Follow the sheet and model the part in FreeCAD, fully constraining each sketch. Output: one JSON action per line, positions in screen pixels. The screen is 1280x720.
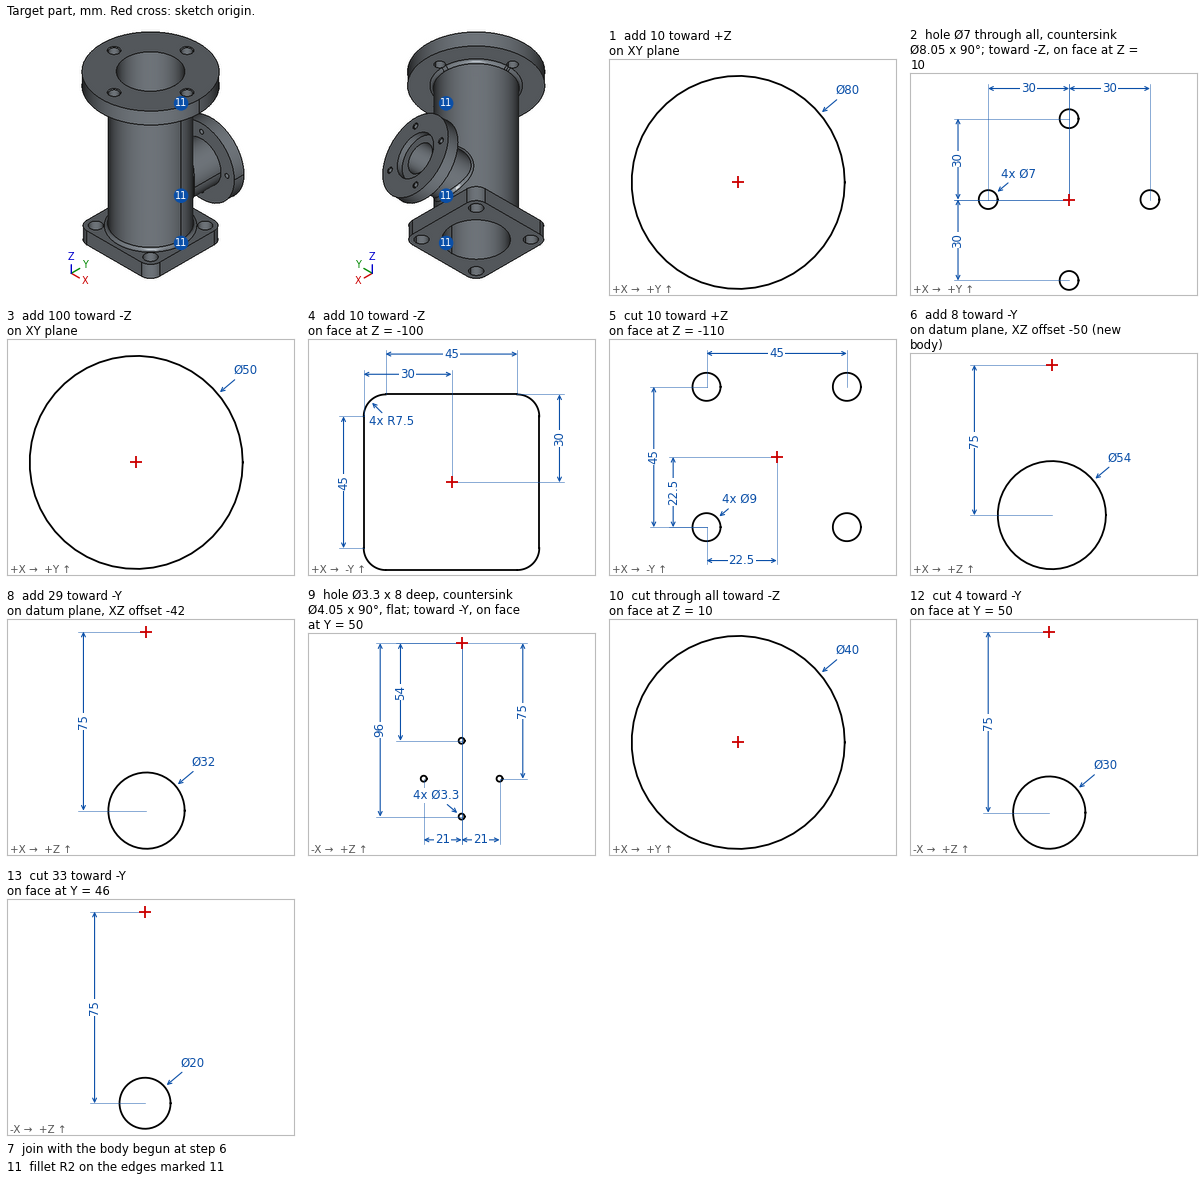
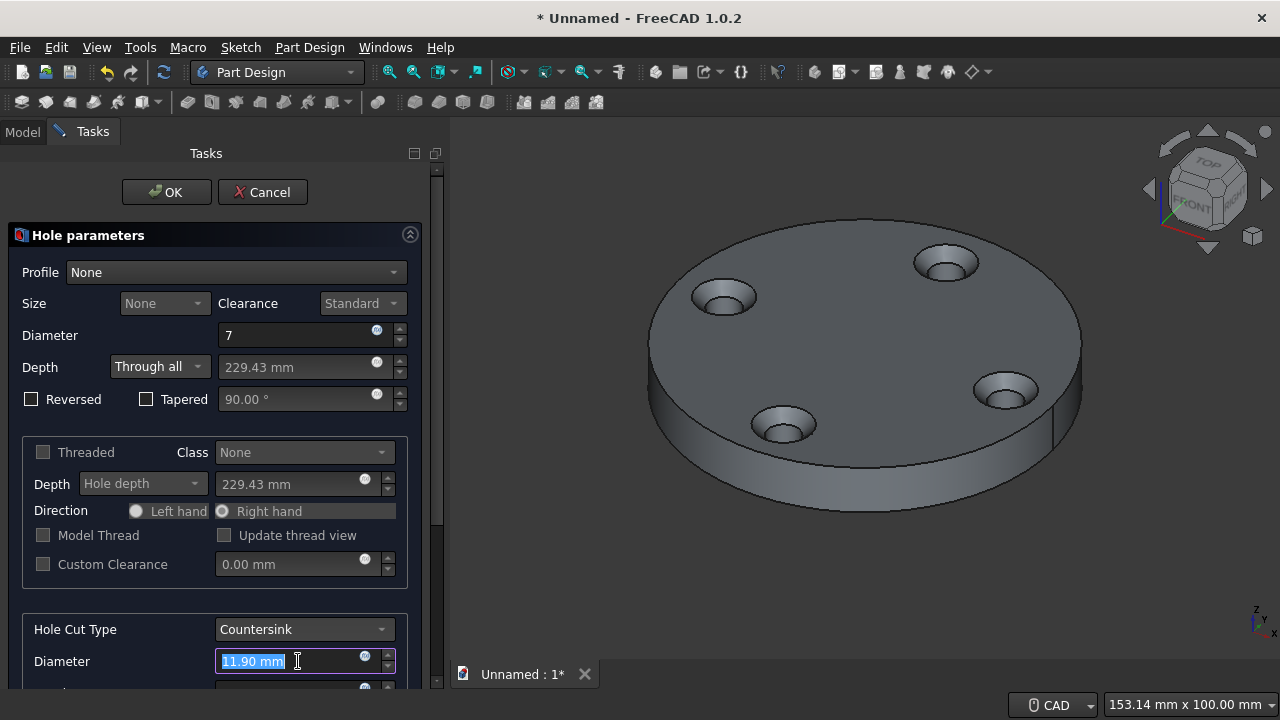
{"action": "type", "text": "8.05"}
{"action": "key", "text": "Tab"}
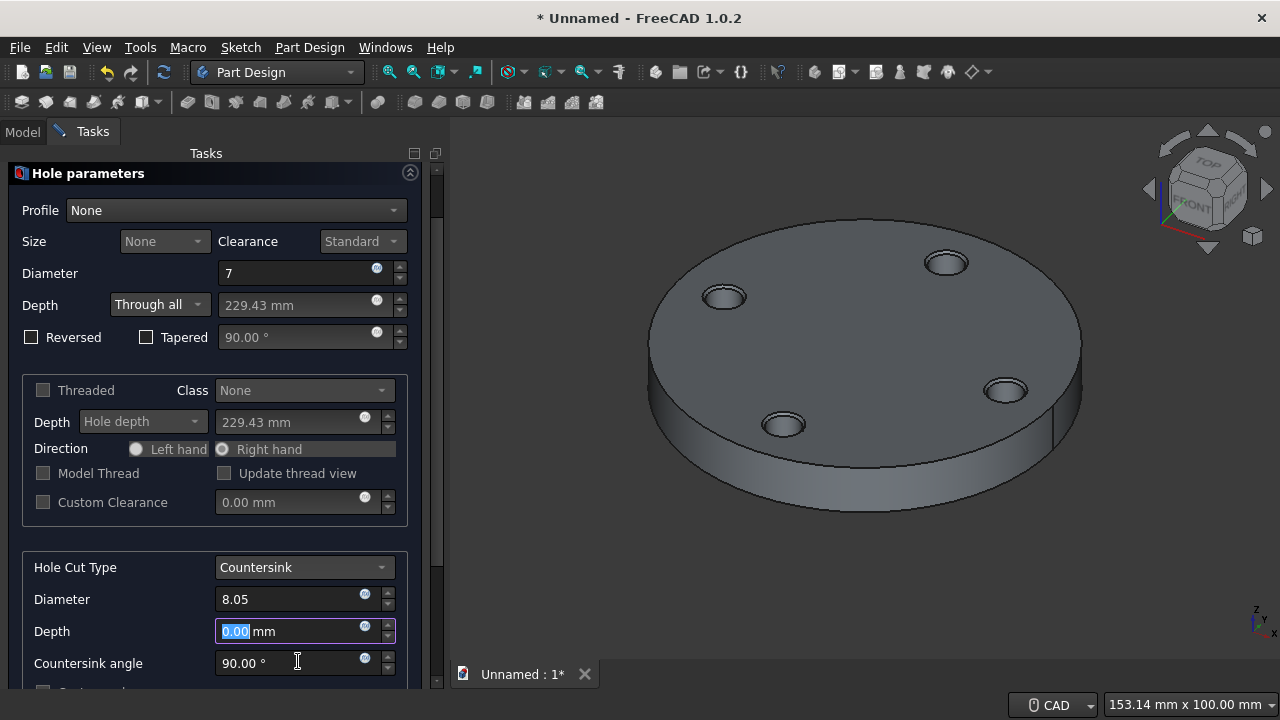
{"action": "scroll", "coordinate": [437, 426], "scroll_direction": "up", "scroll_amount": 2}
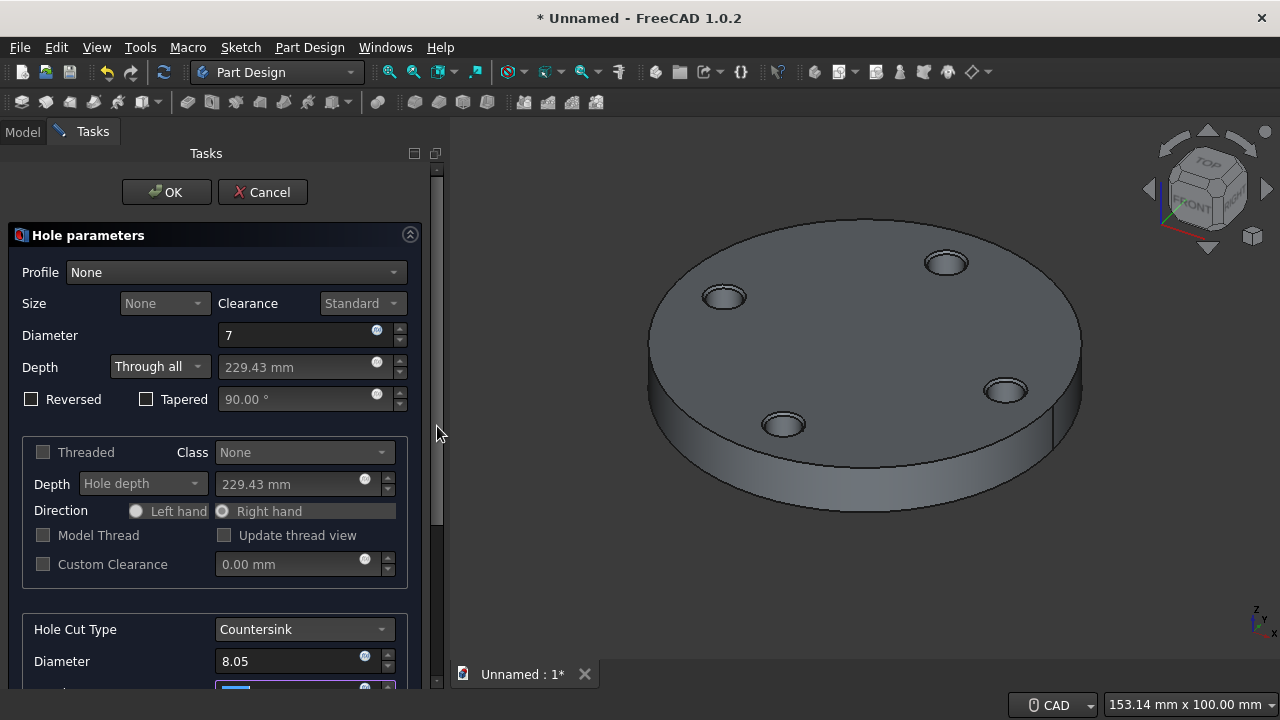
{"action": "left_click", "coordinate": [167, 192]}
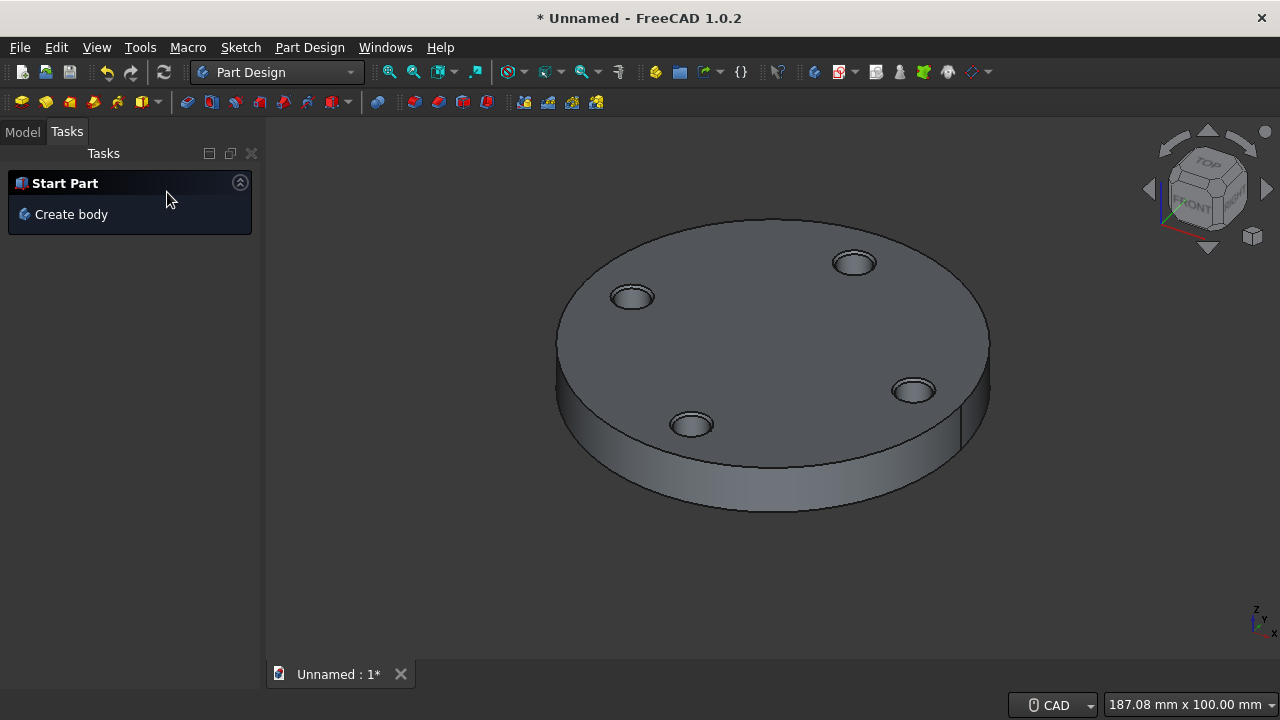
{"action": "left_click", "coordinate": [840, 72]}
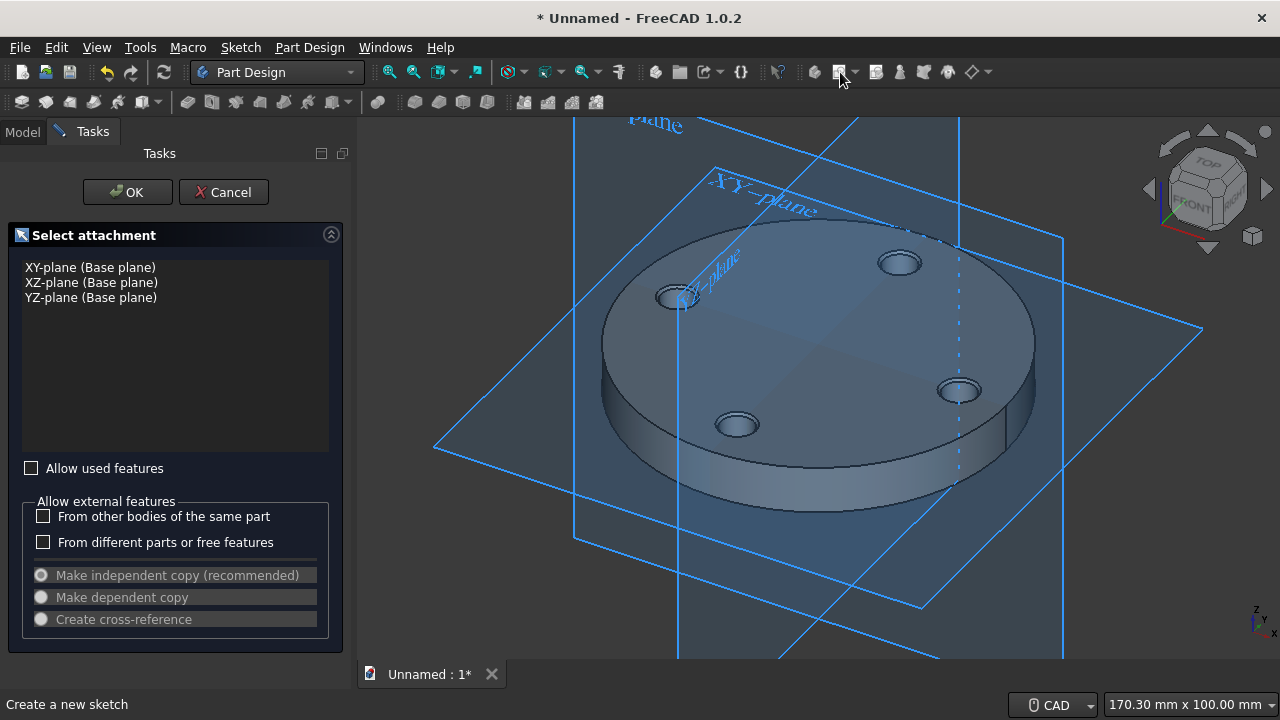
{"action": "left_click", "coordinate": [82, 268]}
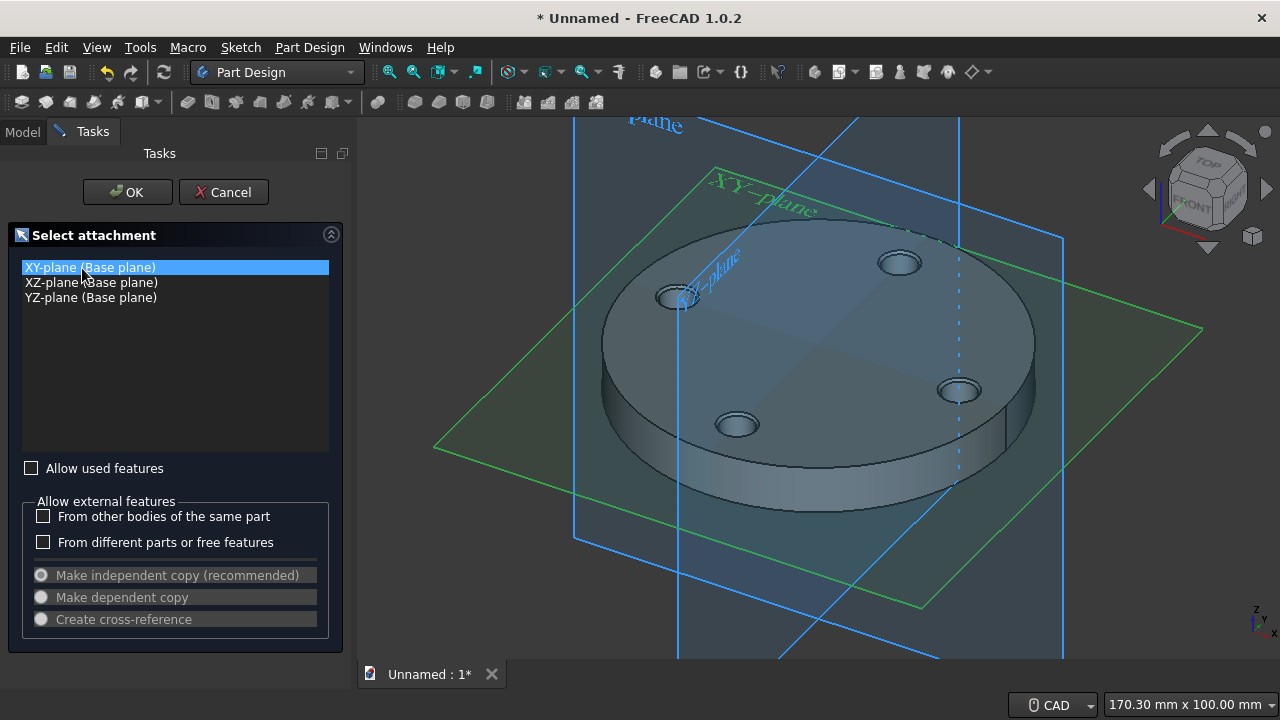
{"action": "left_click", "coordinate": [128, 192]}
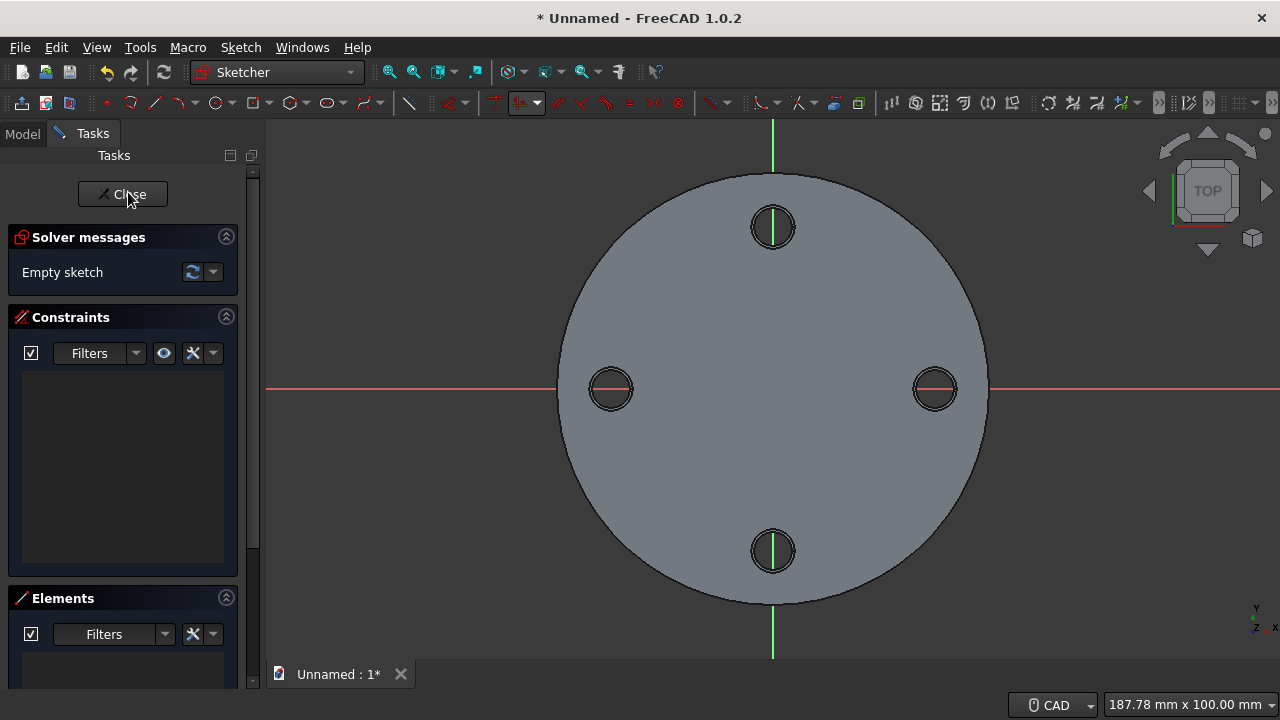
{"action": "left_click", "coordinate": [70, 104]}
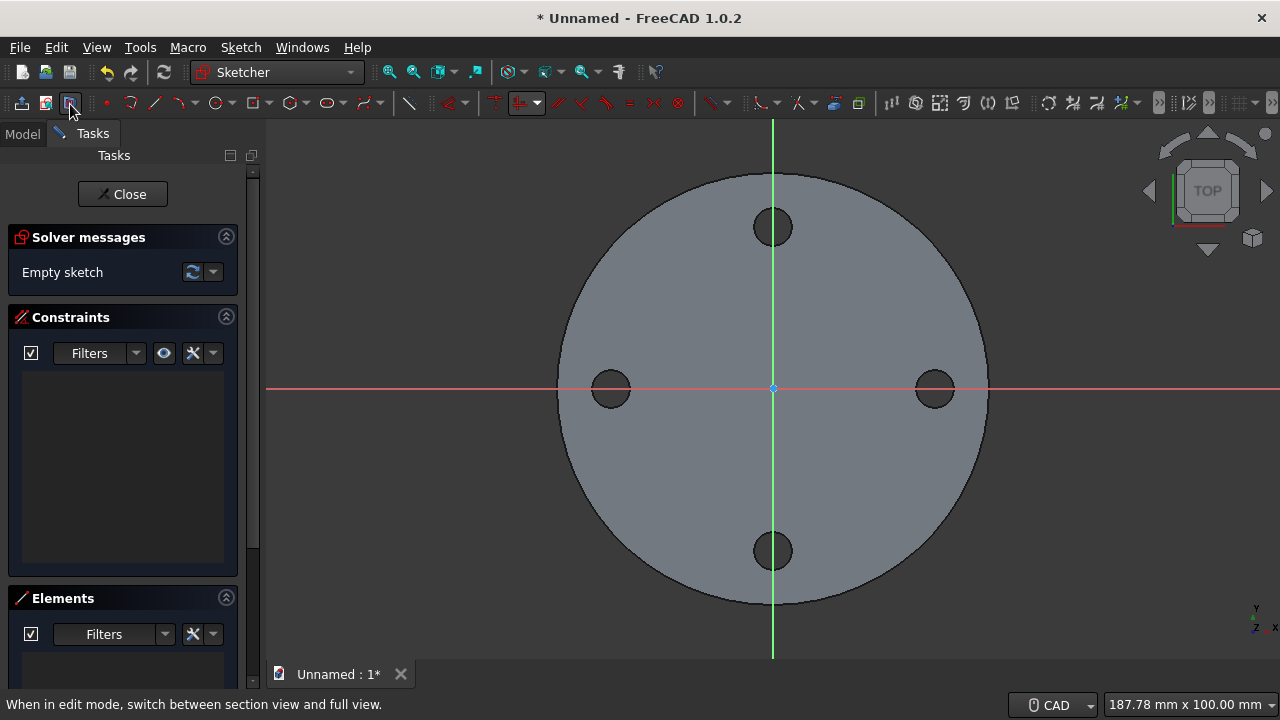
{"action": "left_click", "coordinate": [216, 104]}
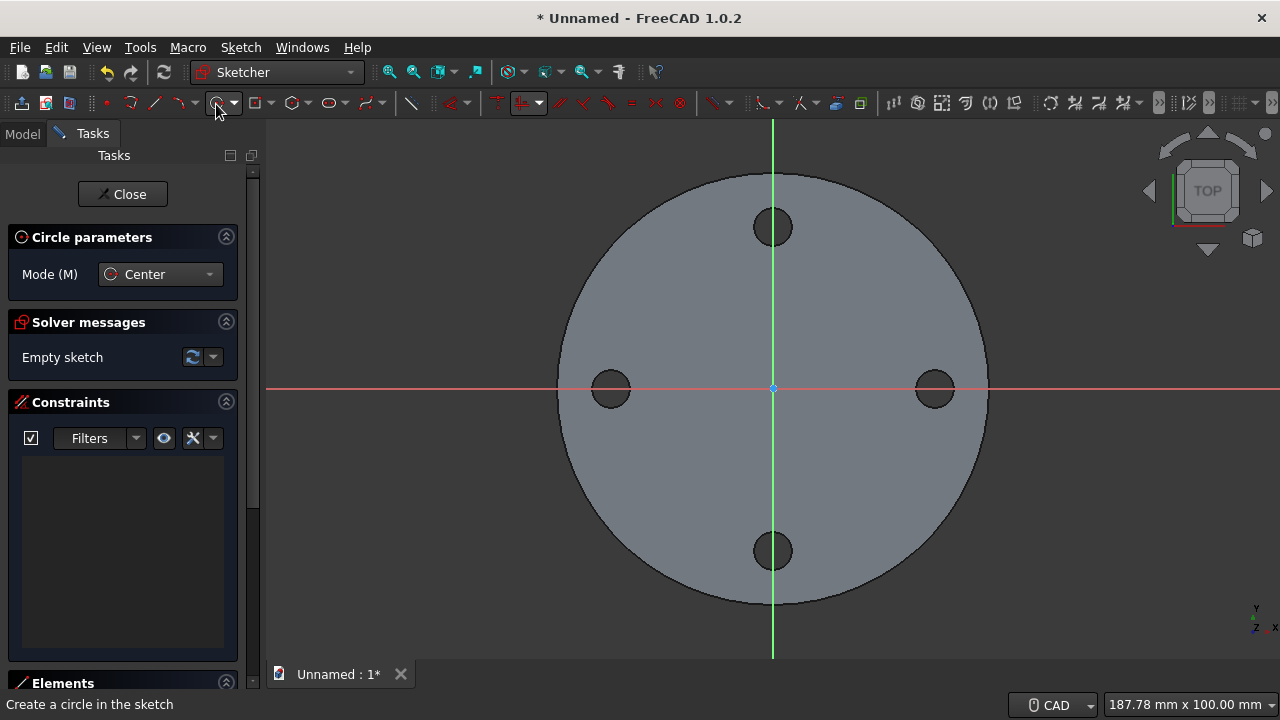
{"action": "left_click", "coordinate": [773, 389]}
{"action": "mouse_move", "coordinate": [868, 294]}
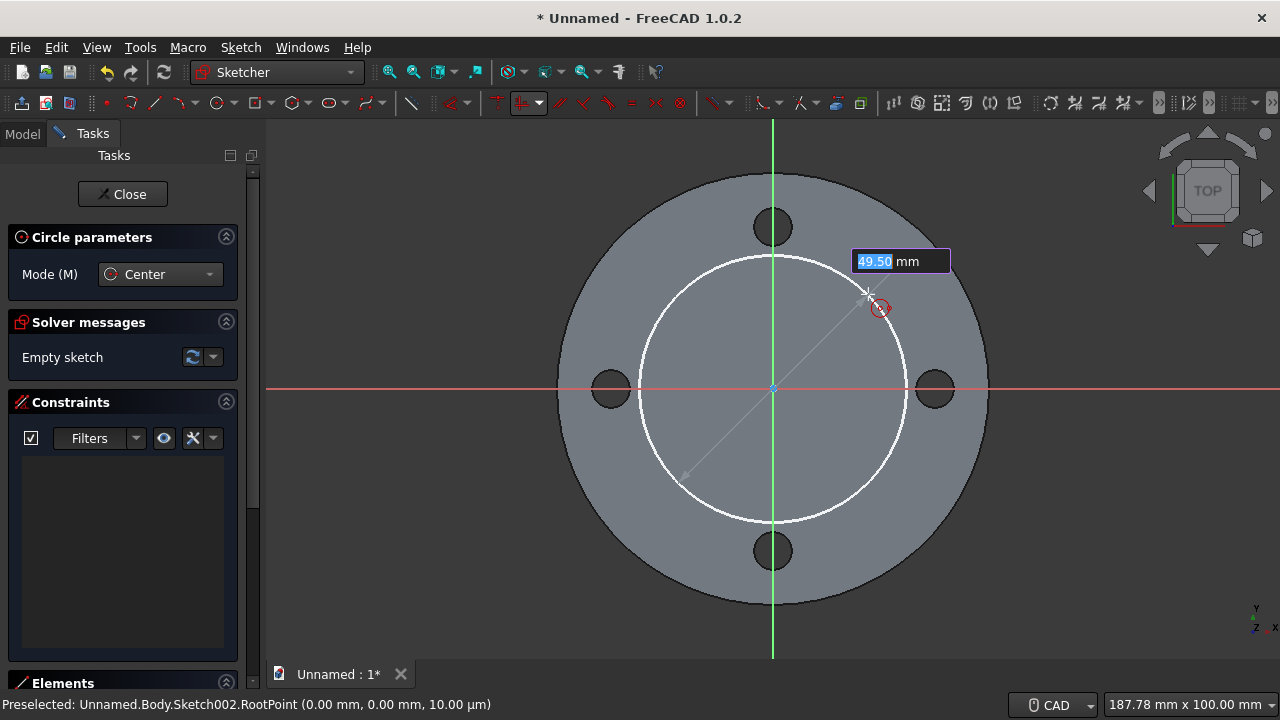
{"action": "type", "text": "50"}
{"action": "key", "text": "Return"}
{"action": "key", "text": "Escape"}